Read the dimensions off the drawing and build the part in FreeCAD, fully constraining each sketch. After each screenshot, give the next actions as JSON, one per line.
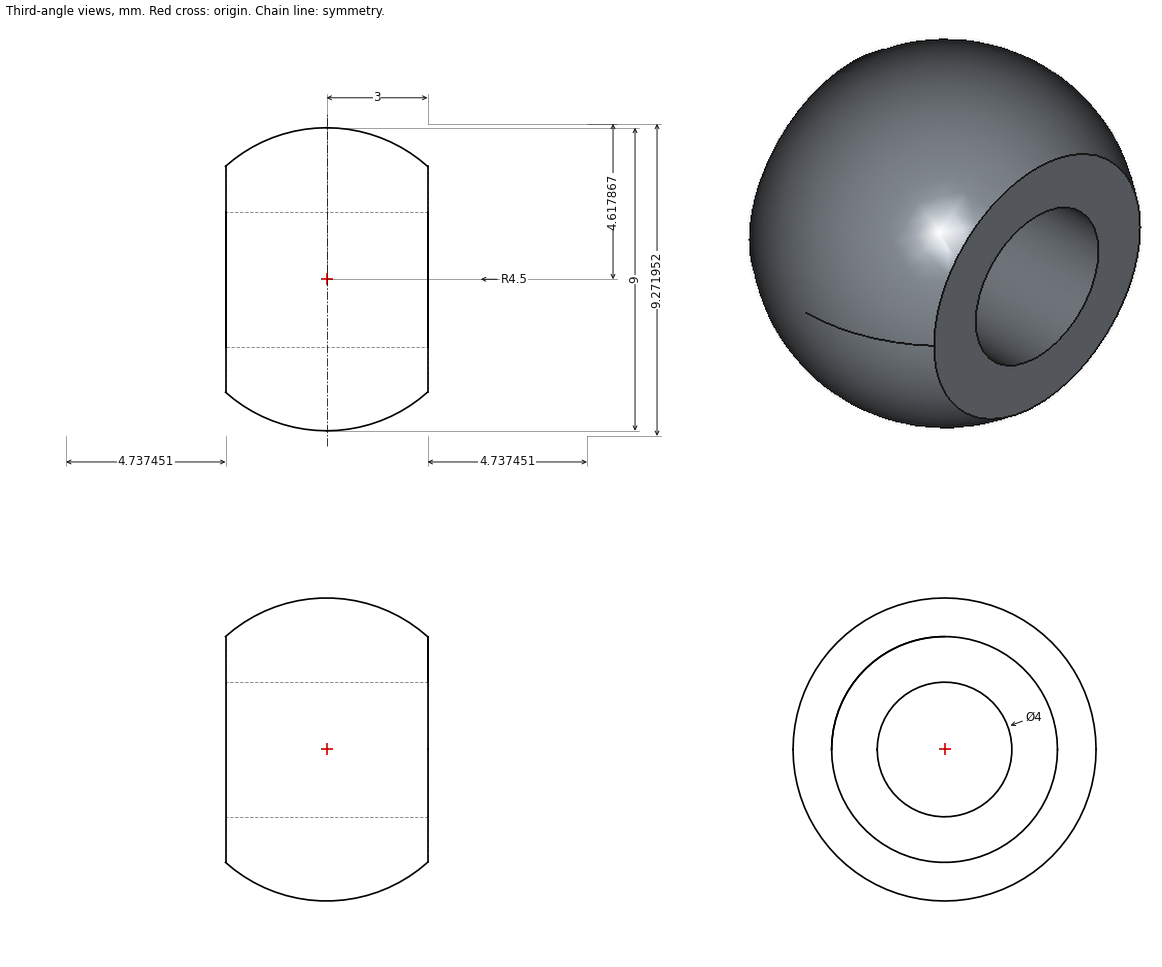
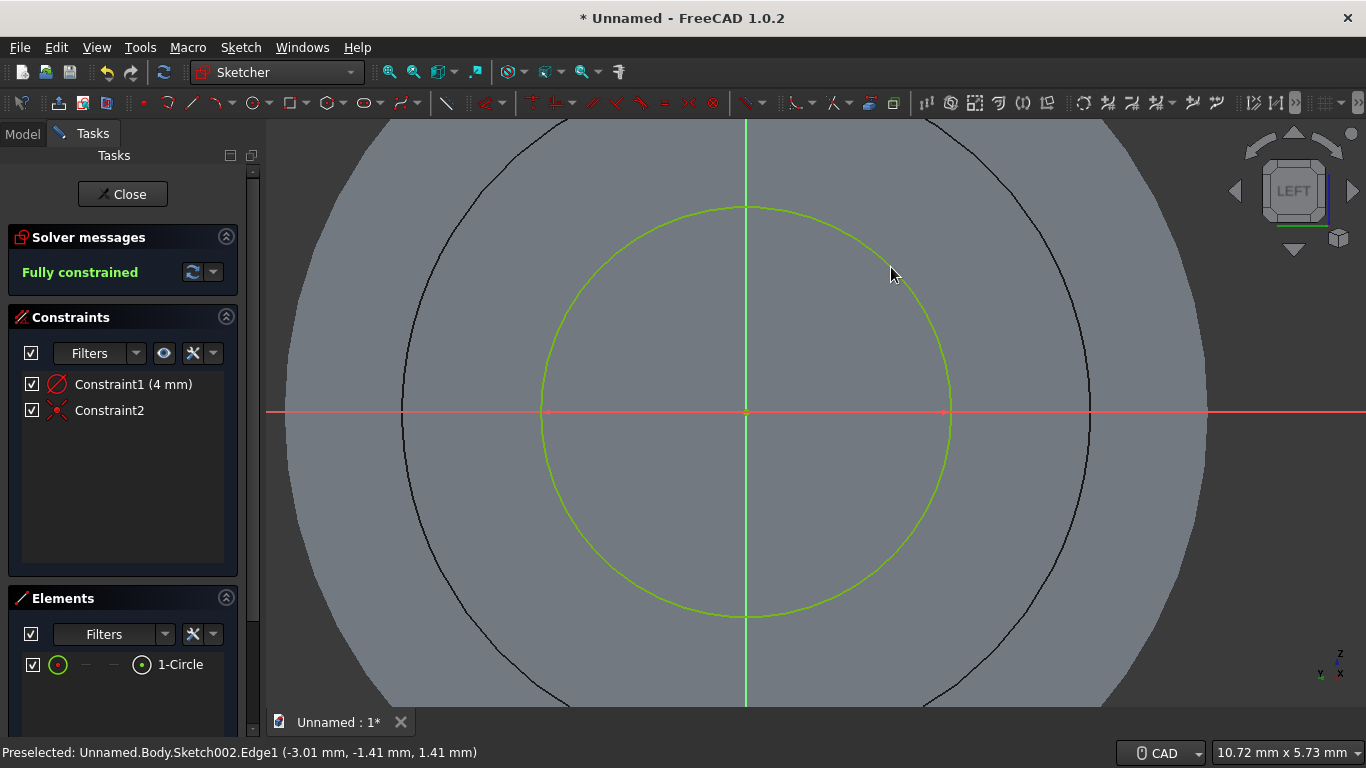
{"action": "left_click", "coordinate": [123, 194]}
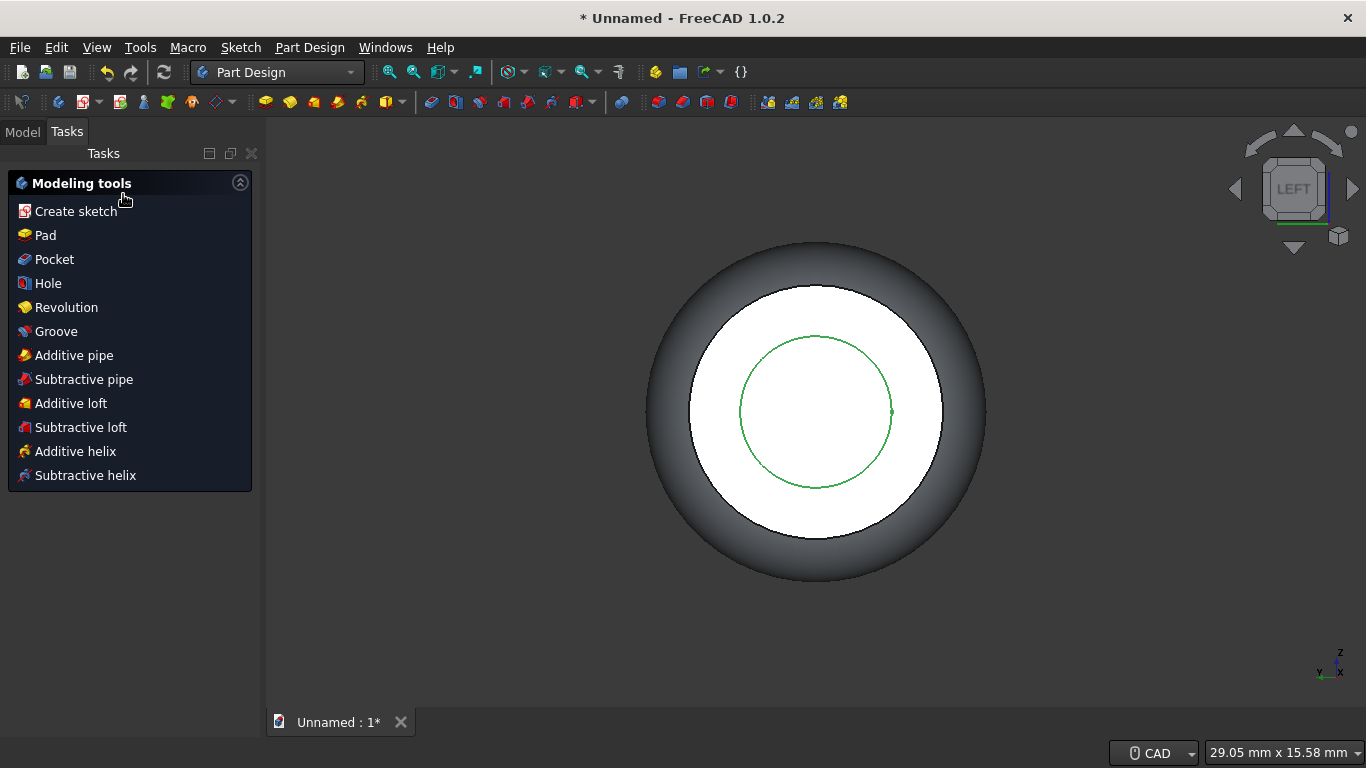
{"action": "left_click", "coordinate": [432, 102]}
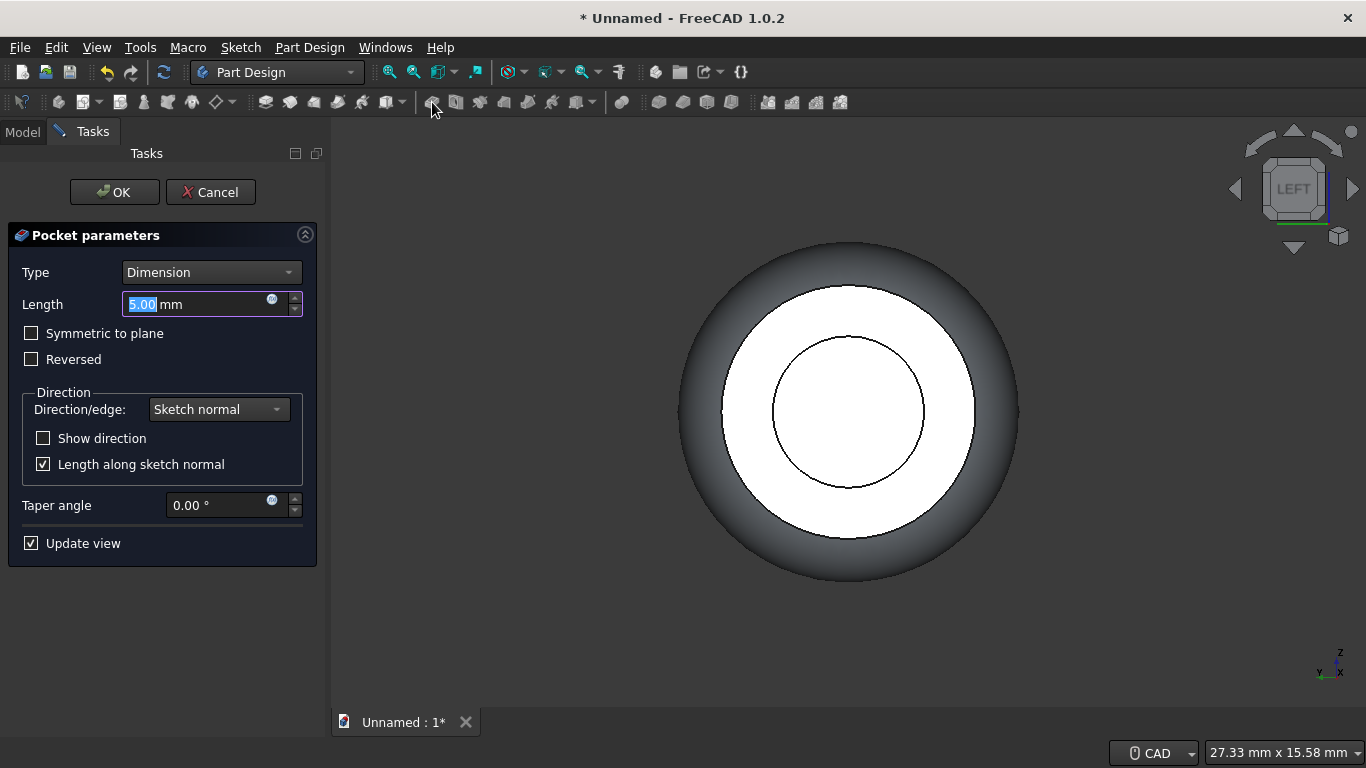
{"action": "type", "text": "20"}
{"action": "key", "text": "Tab"}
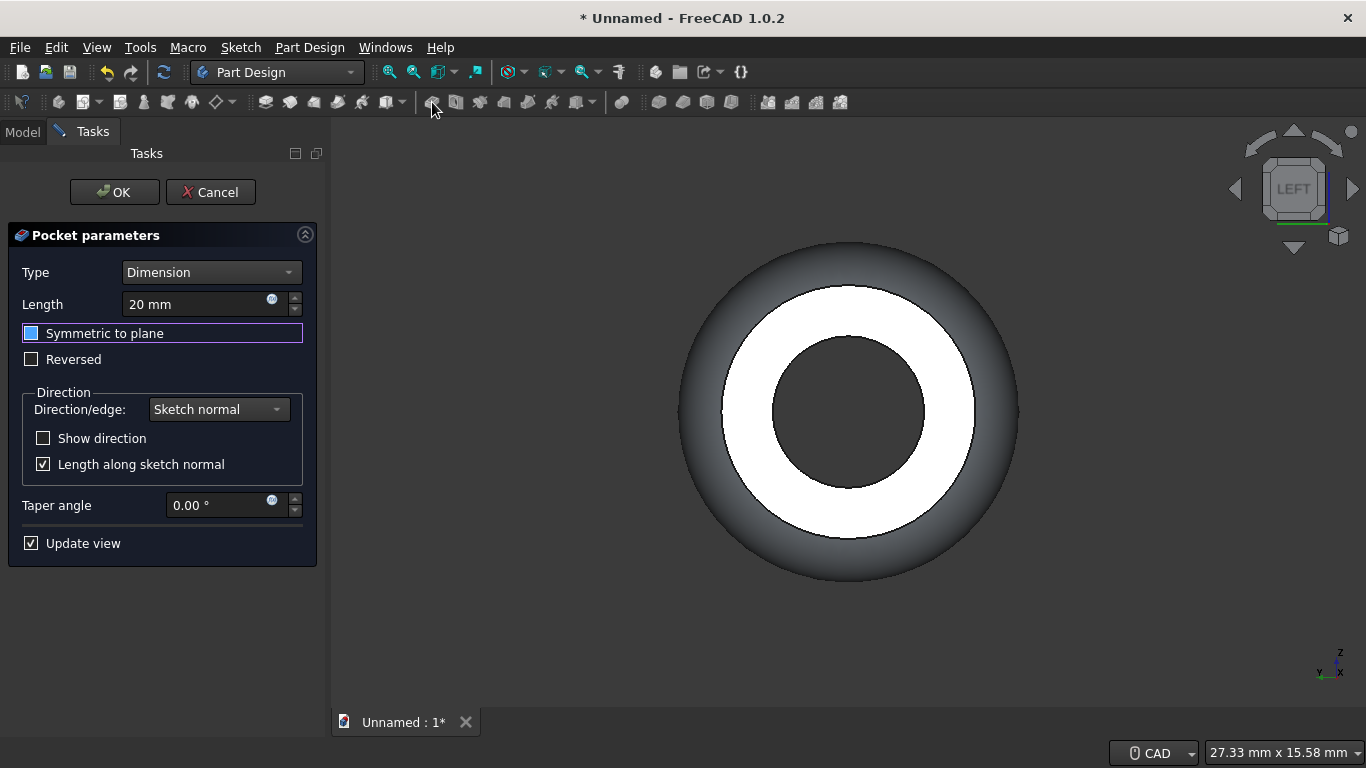
{"action": "left_click", "coordinate": [115, 192]}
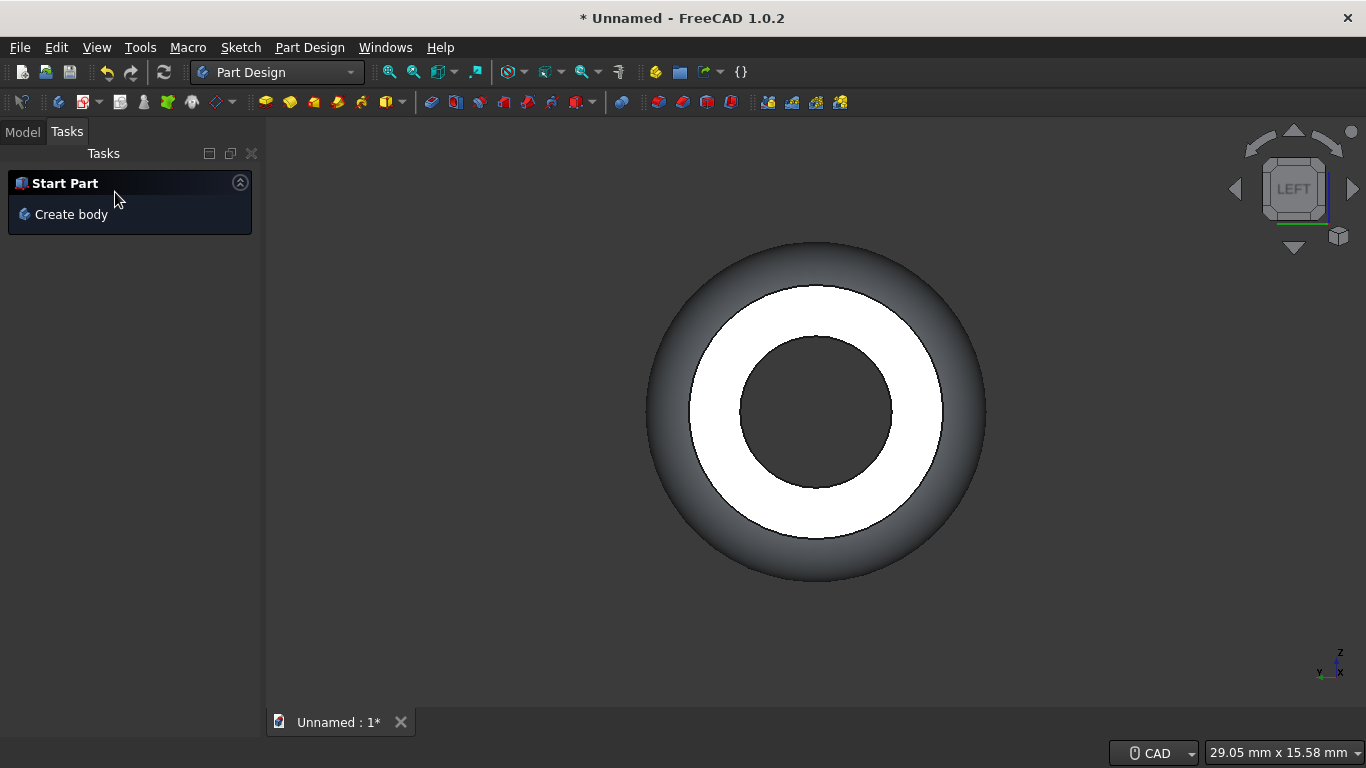
{"action": "key", "text": "0"}